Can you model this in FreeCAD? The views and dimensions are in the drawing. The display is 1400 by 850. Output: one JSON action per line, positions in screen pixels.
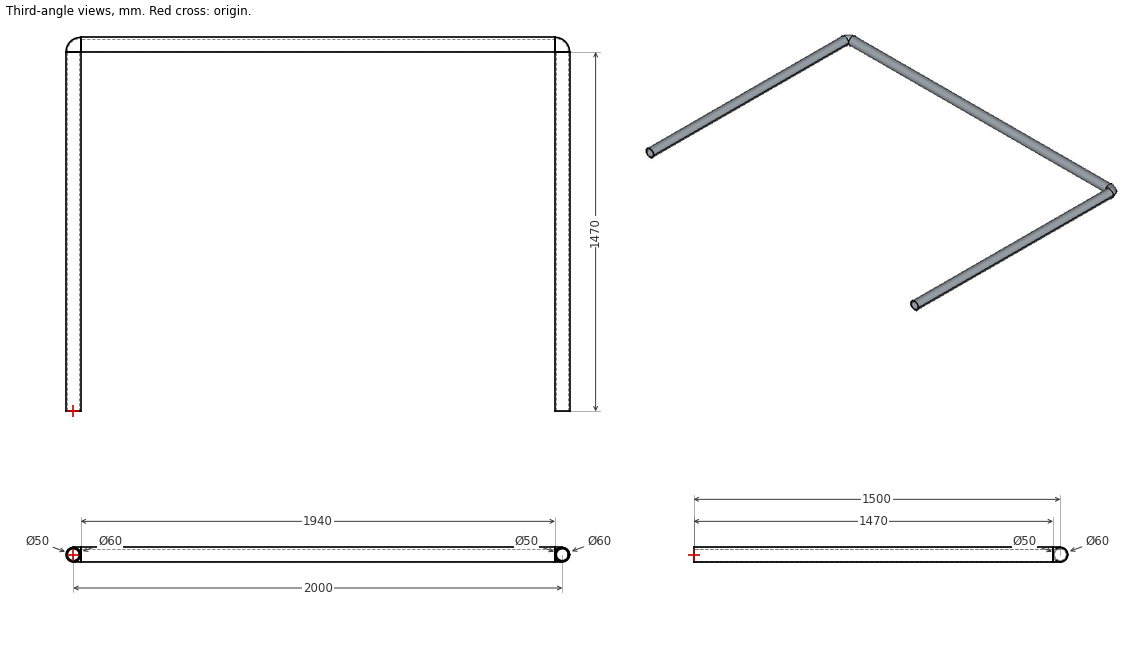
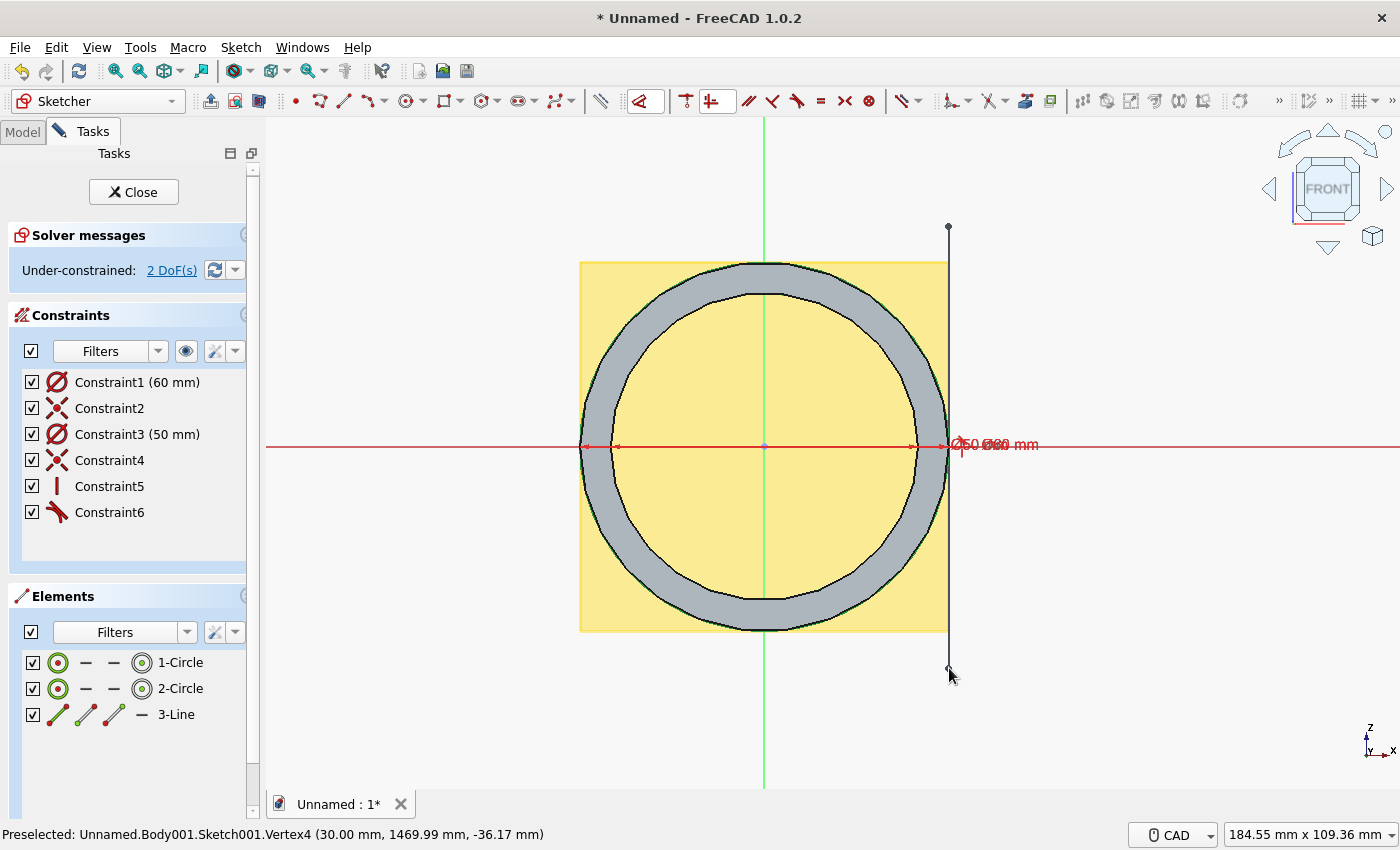
{"action": "left_click", "coordinate": [949, 360]}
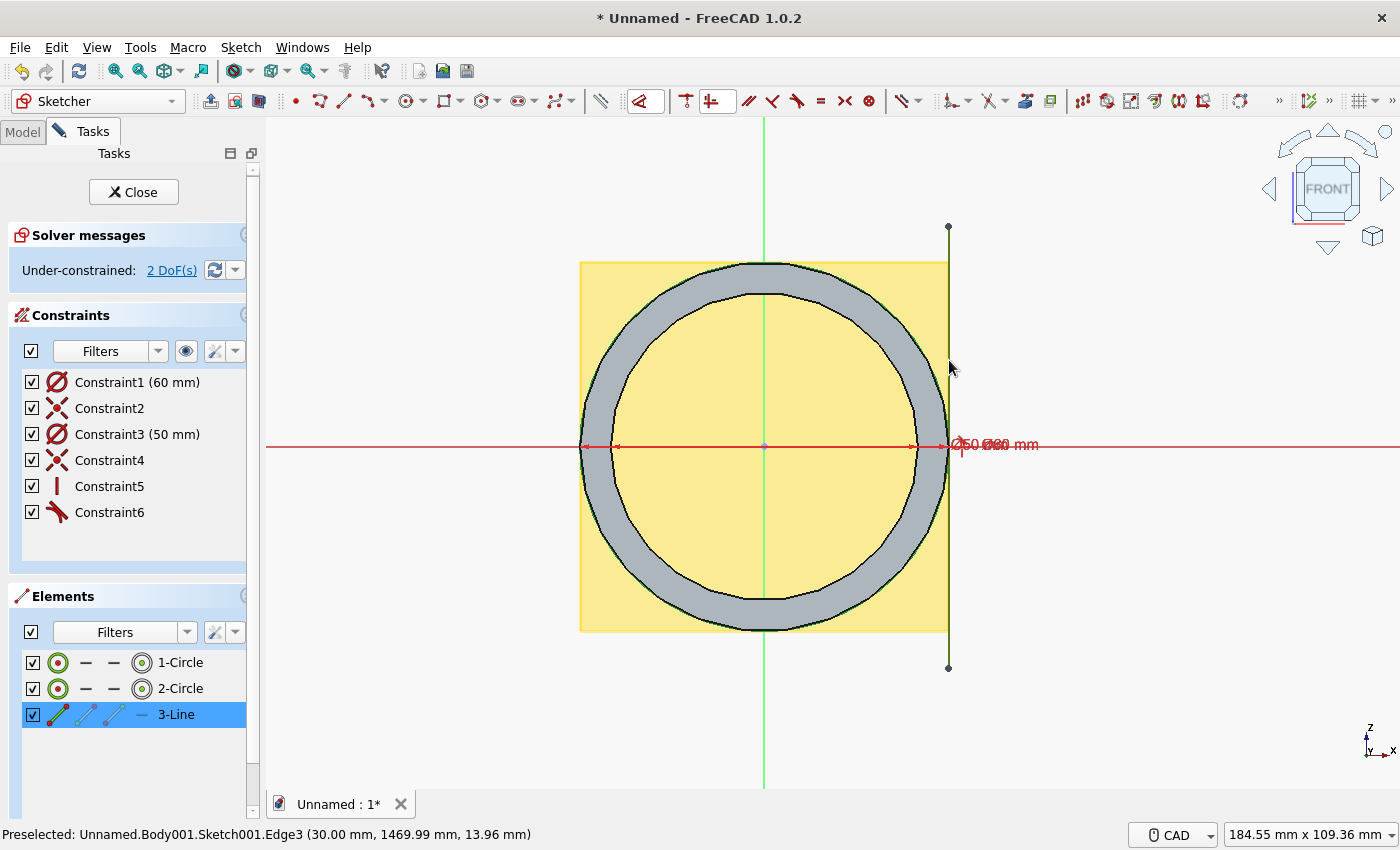
{"action": "left_click", "coordinate": [602, 102]}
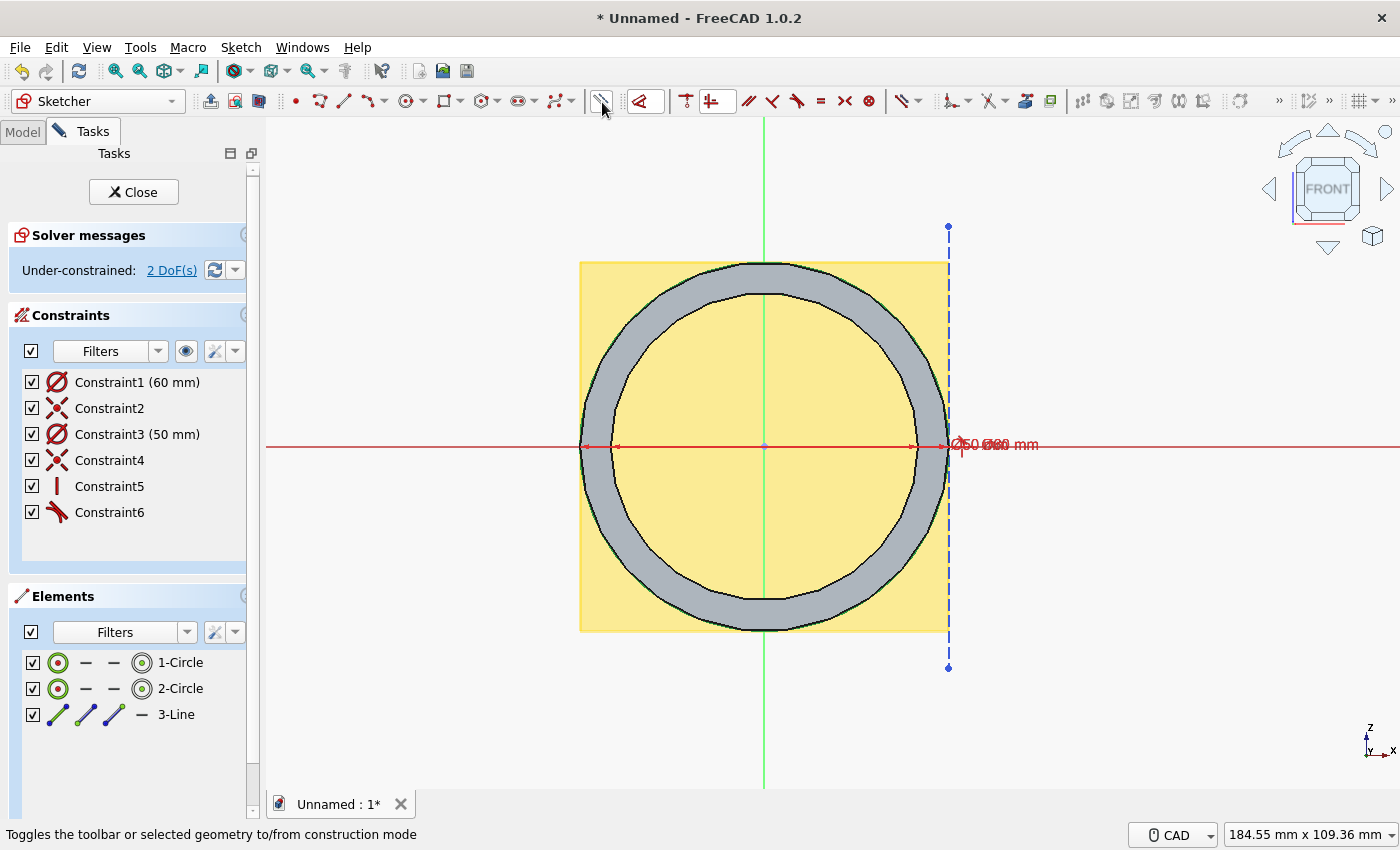
{"action": "left_click", "coordinate": [134, 192]}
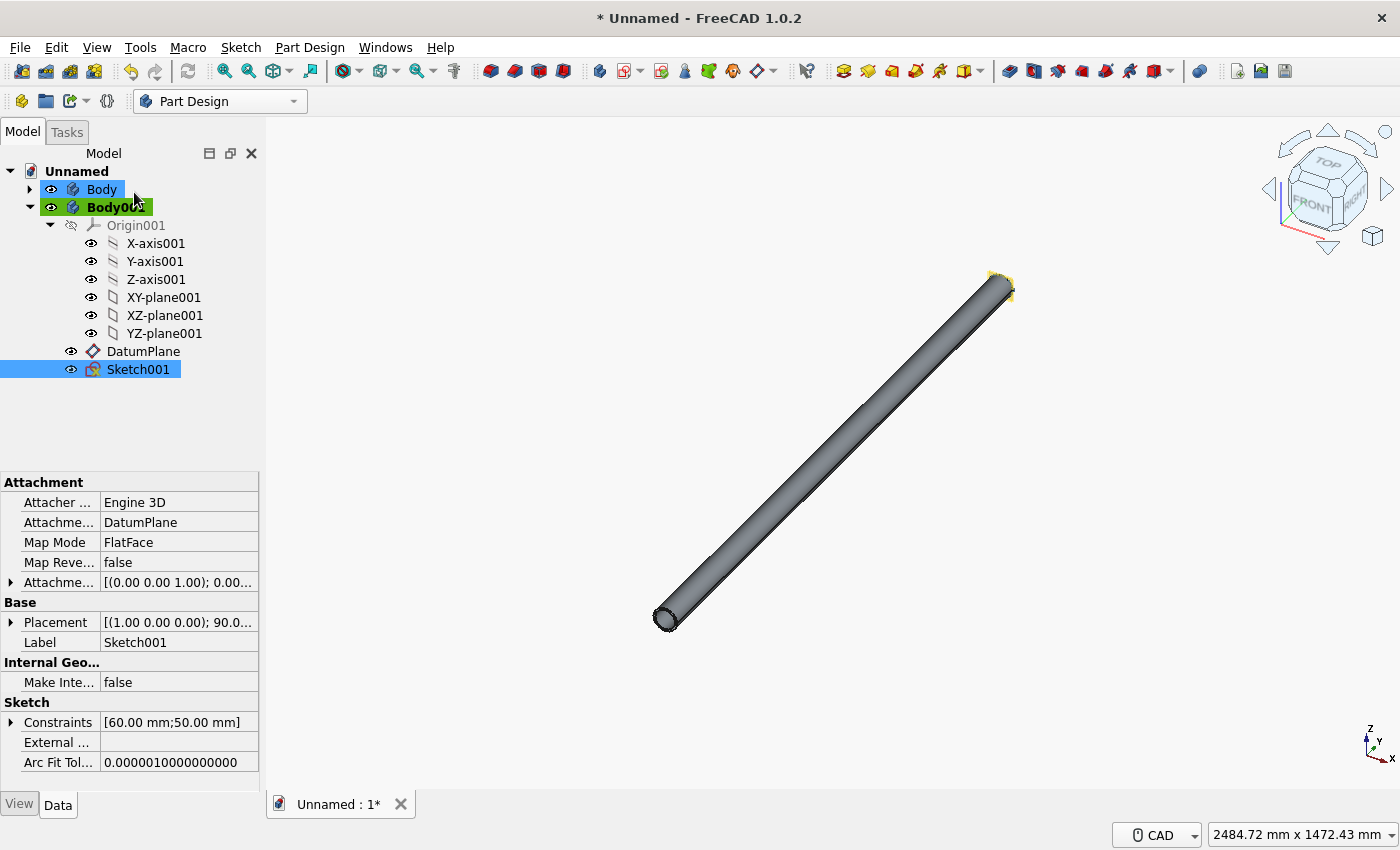
{"action": "left_click", "coordinate": [868, 72]}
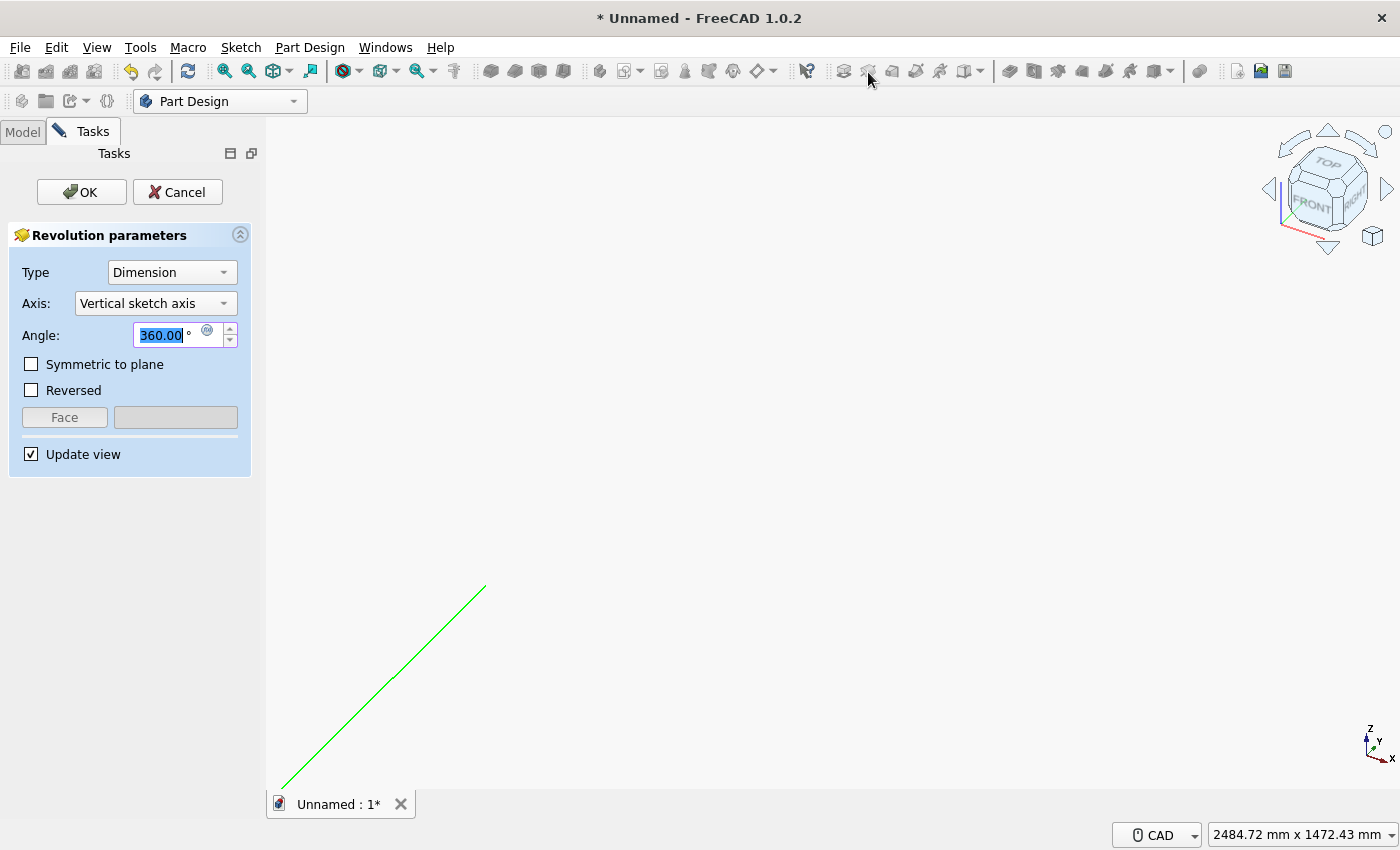
{"action": "left_click", "coordinate": [156, 304]}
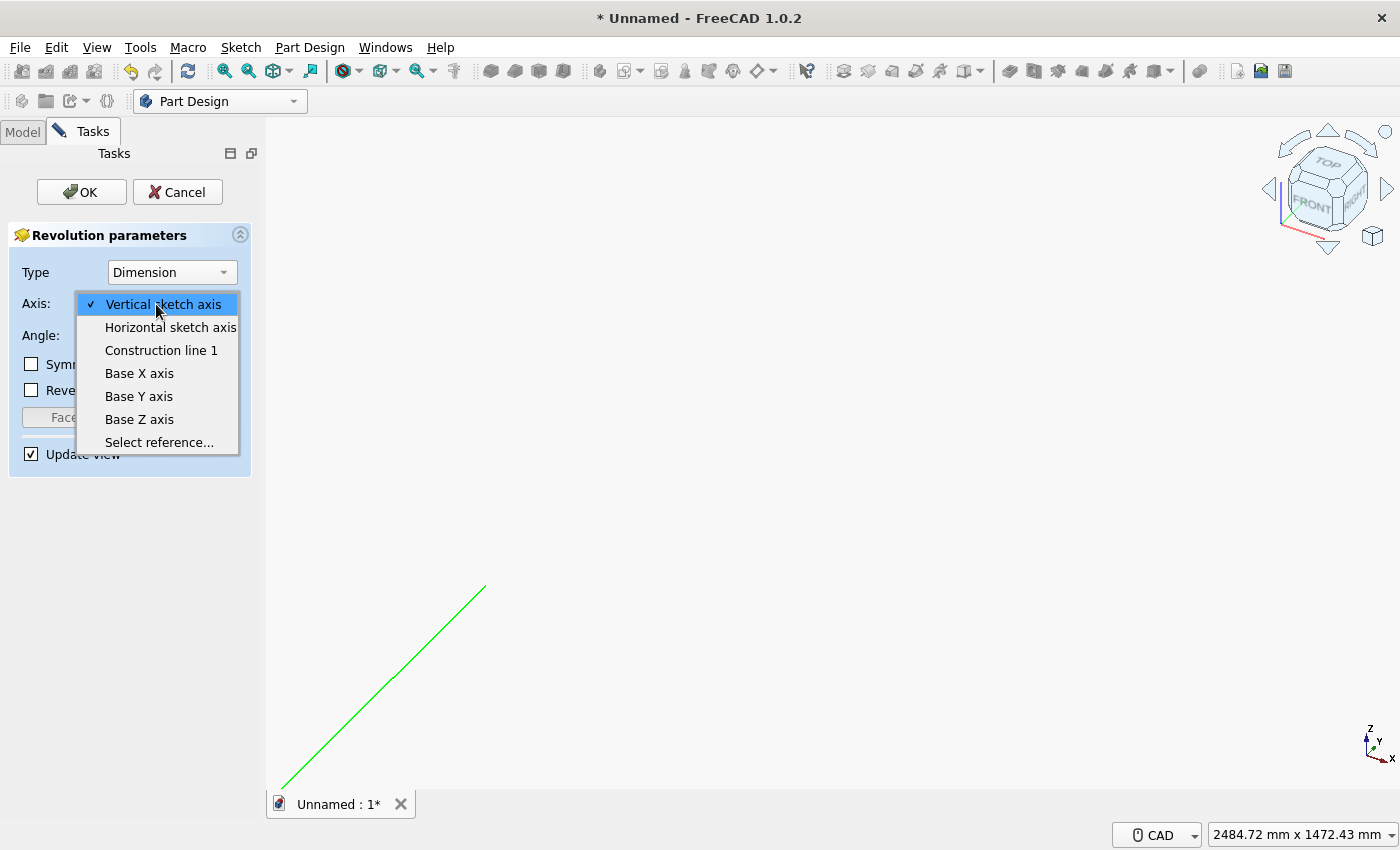
{"action": "left_click", "coordinate": [156, 350]}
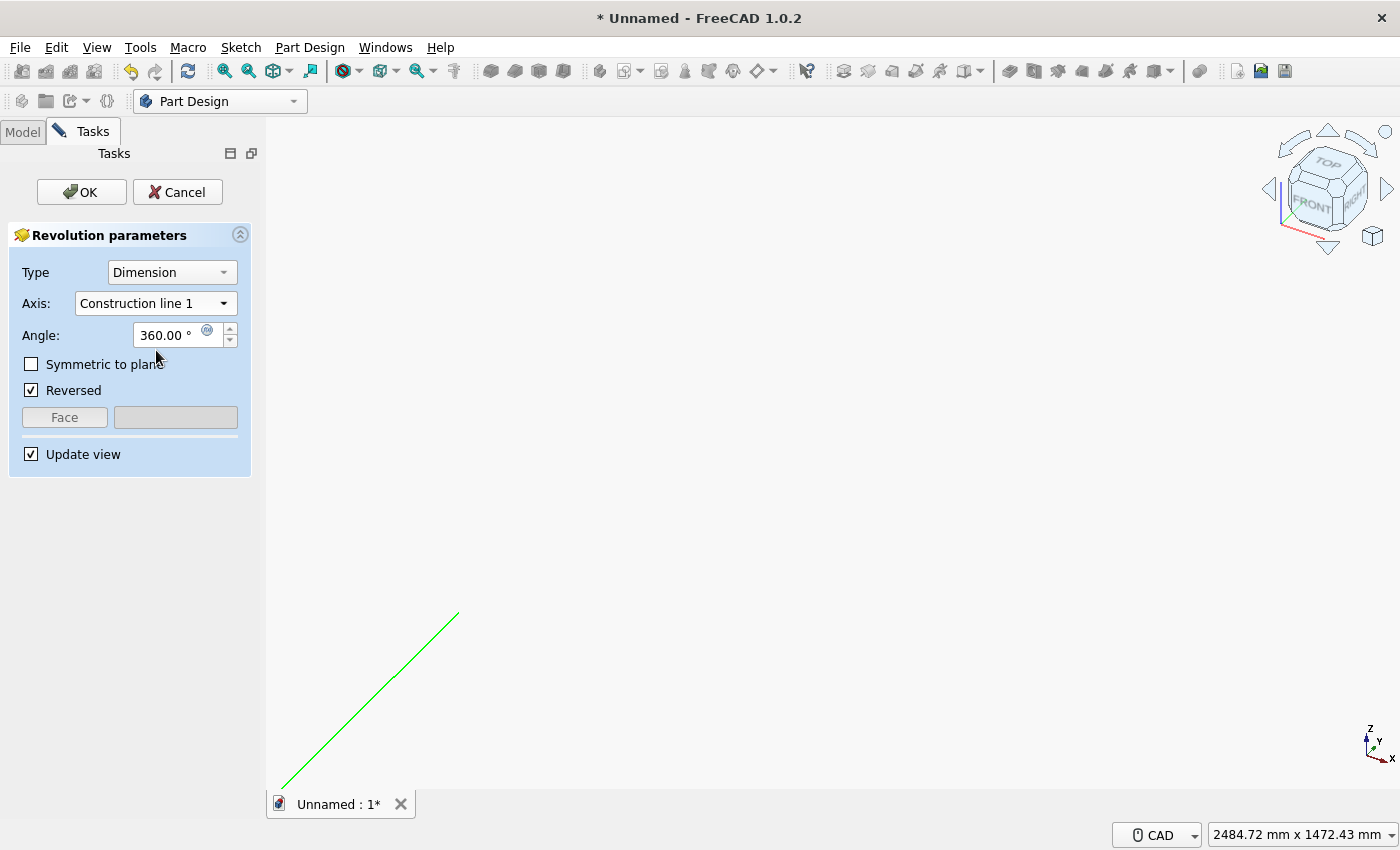
{"action": "triple_click", "coordinate": [178, 335]}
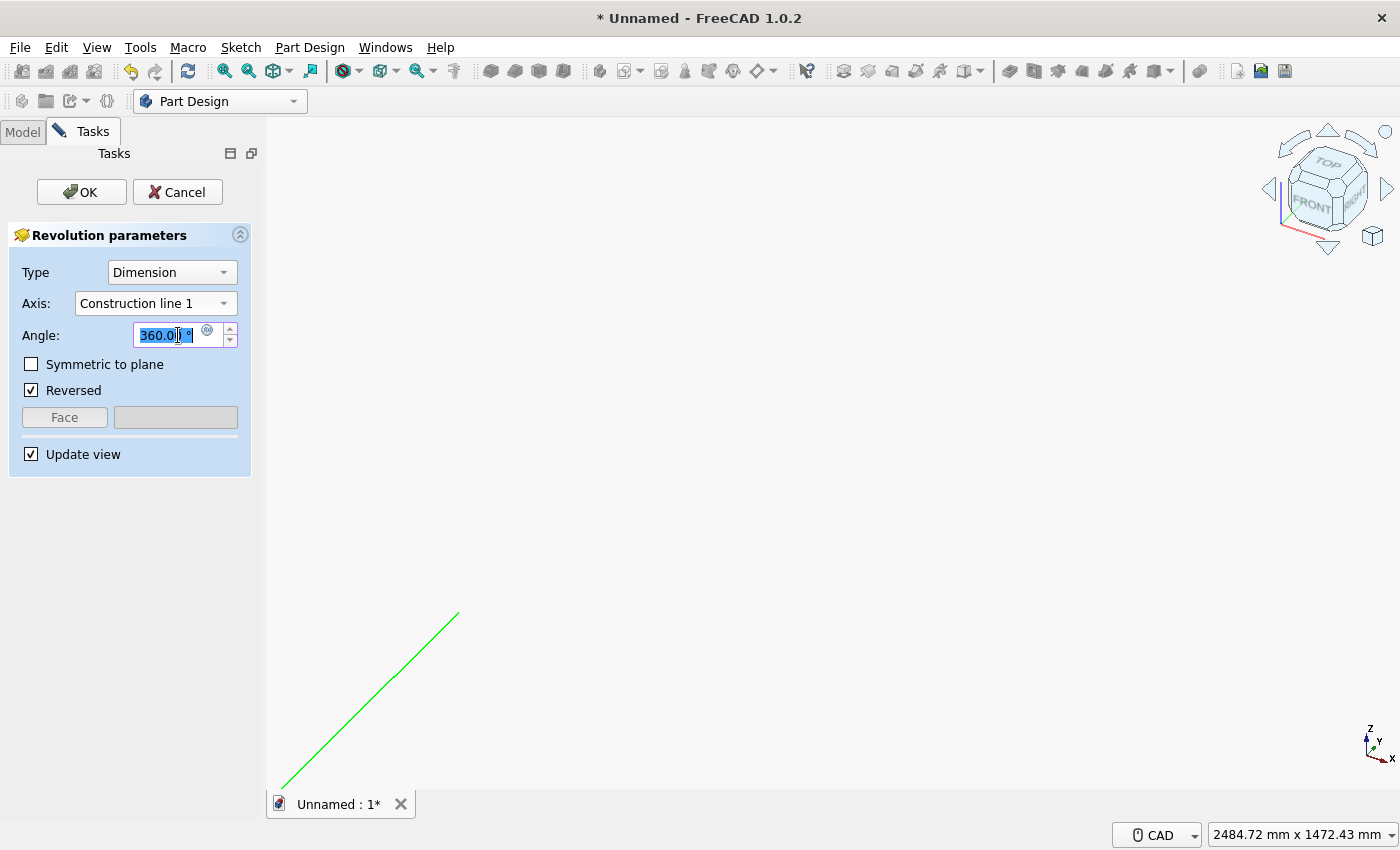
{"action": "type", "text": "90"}
{"action": "key", "text": "Tab"}